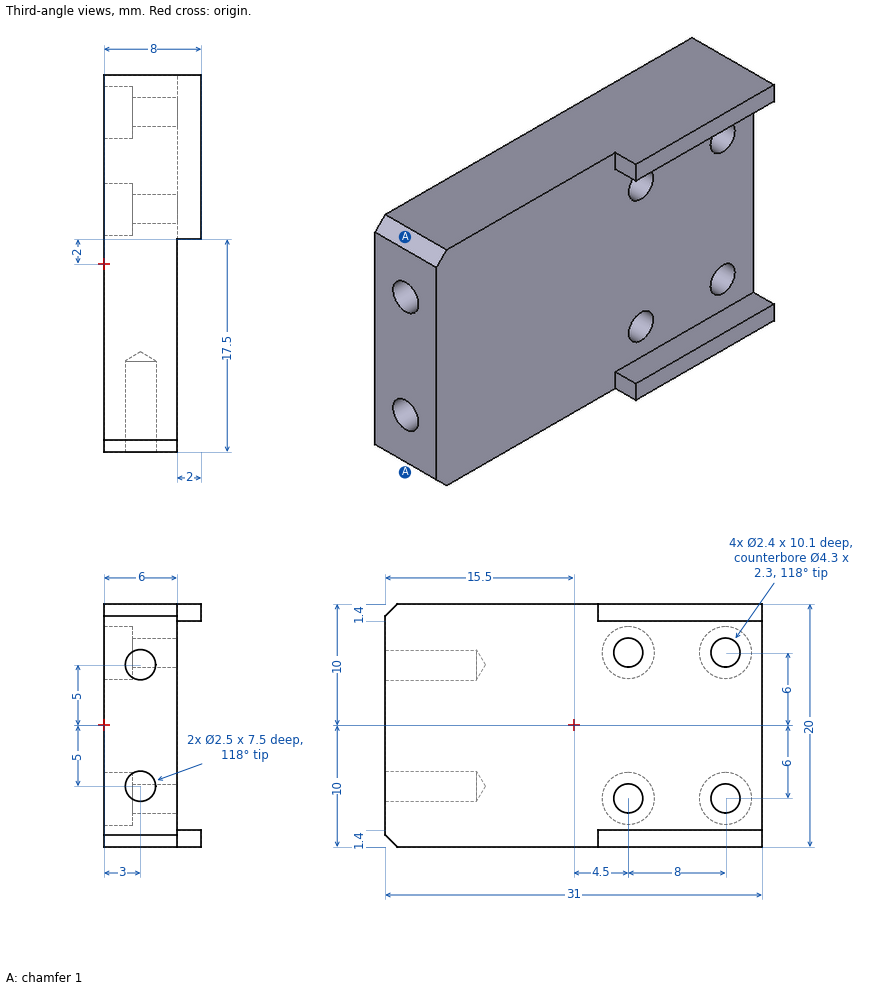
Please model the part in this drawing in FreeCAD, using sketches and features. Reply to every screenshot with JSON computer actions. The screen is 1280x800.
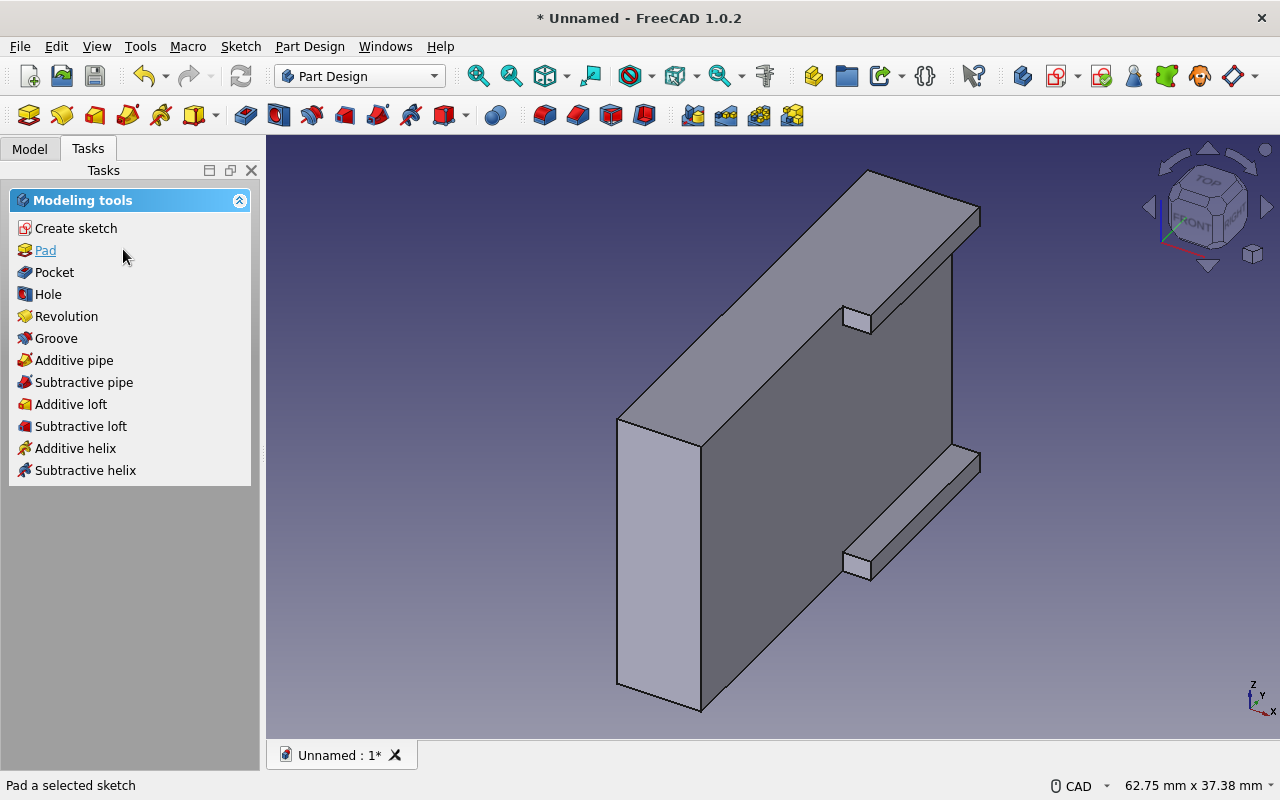
{"action": "left_click", "coordinate": [279, 116]}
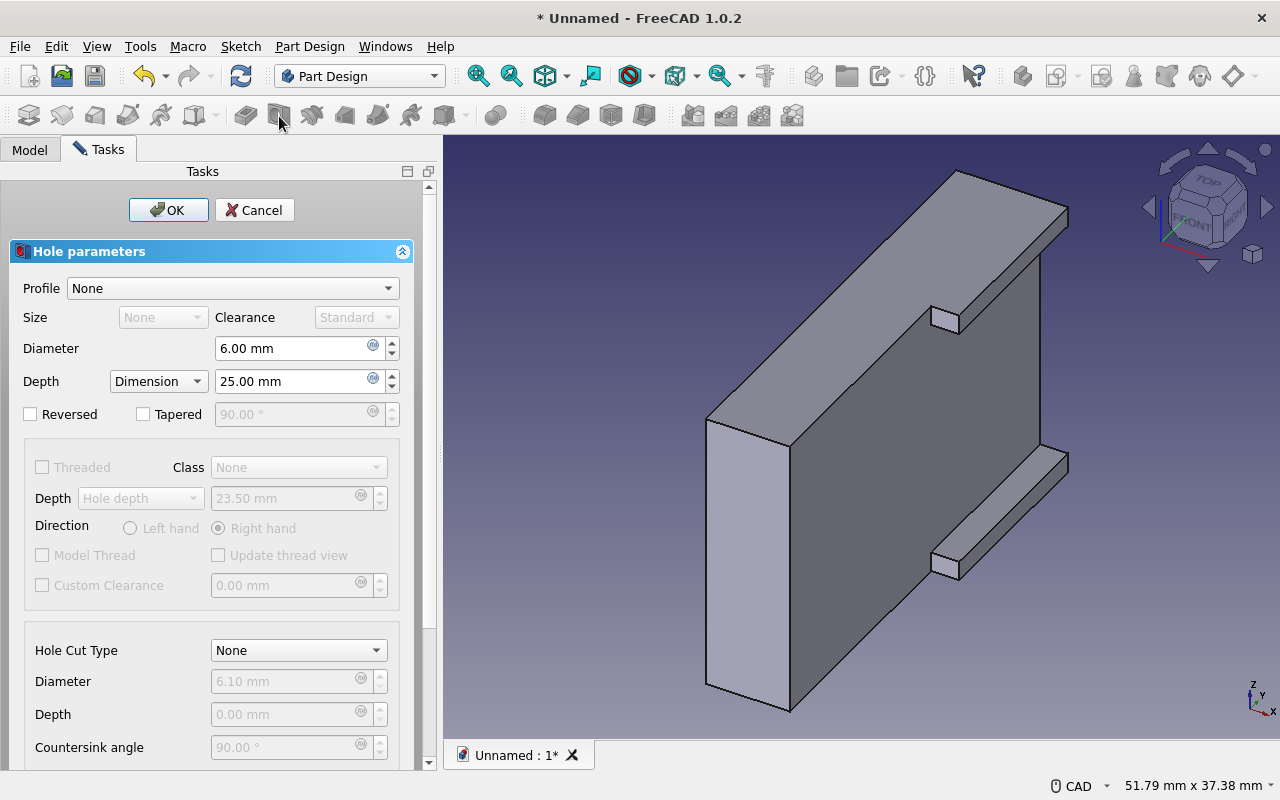
{"action": "triple_click", "coordinate": [300, 348]}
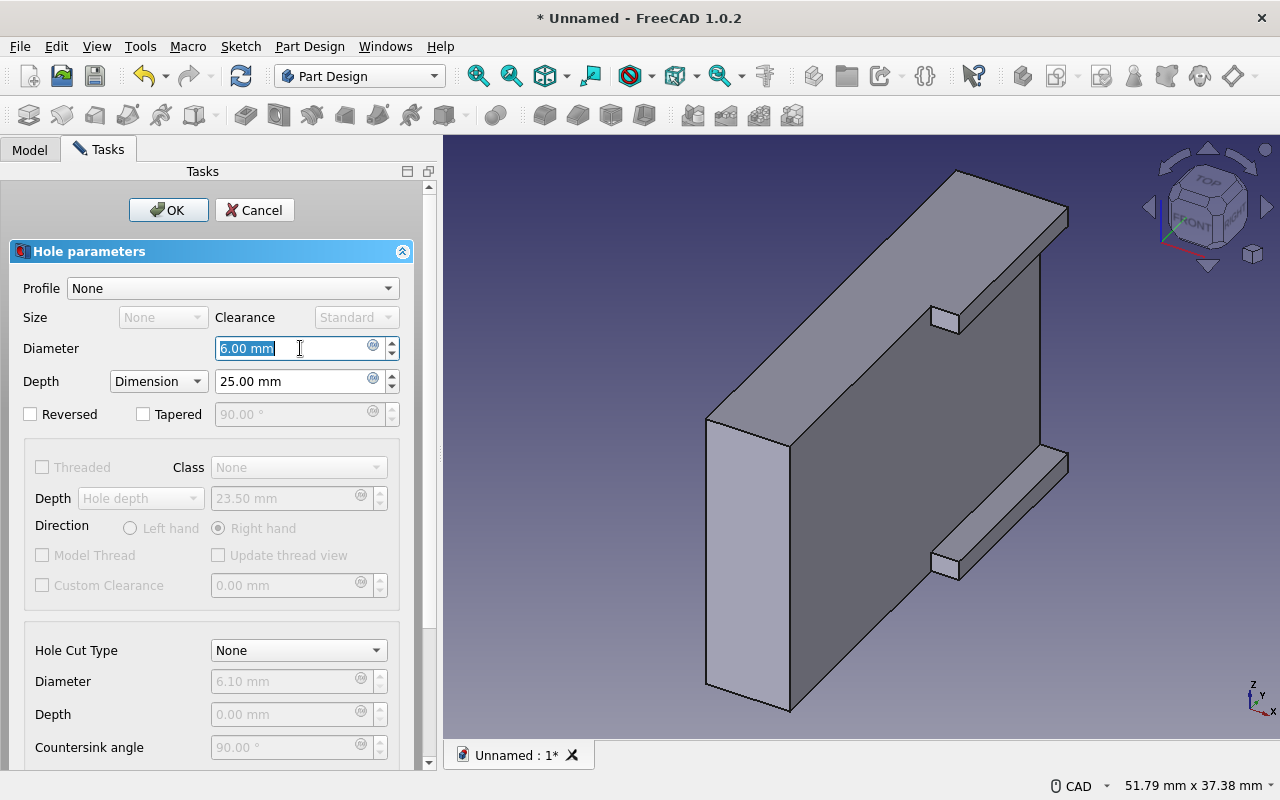
{"action": "type", "text": "2.4"}
{"action": "key", "text": "Tab"}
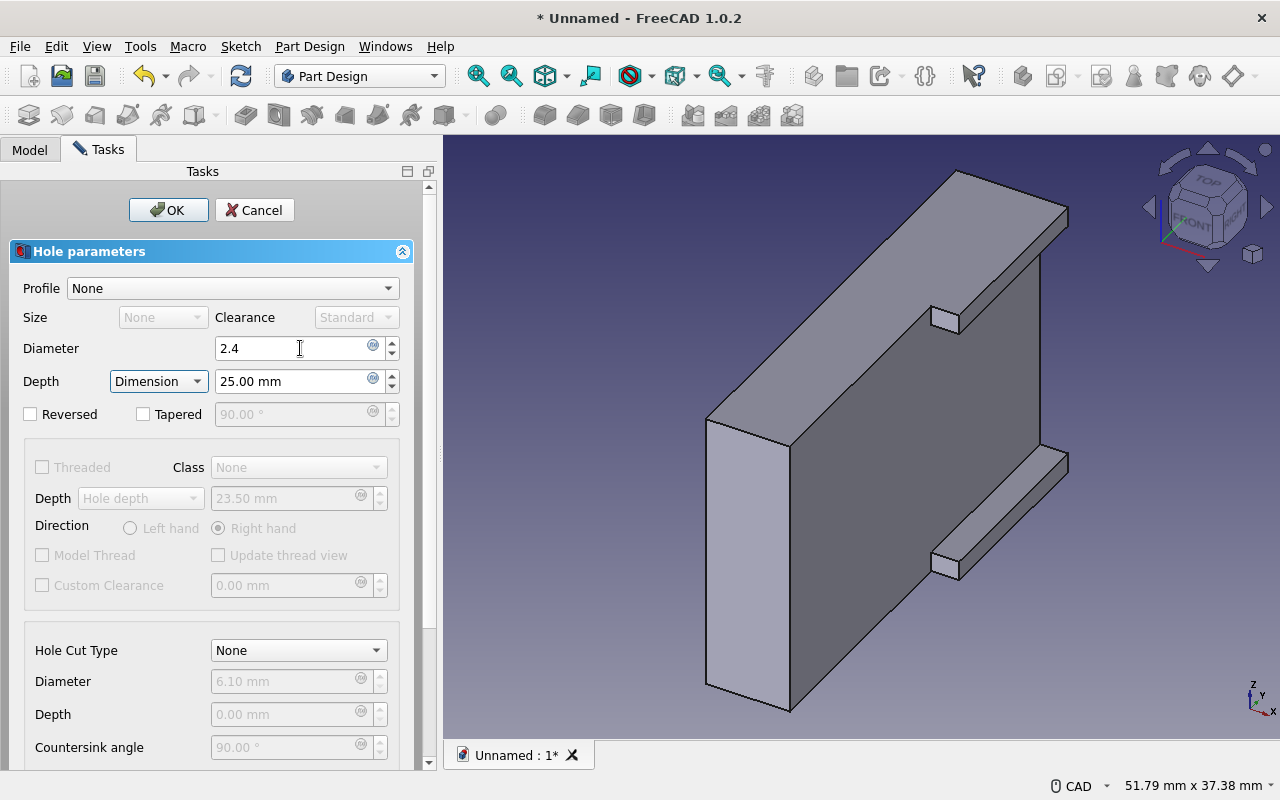
{"action": "triple_click", "coordinate": [300, 382]}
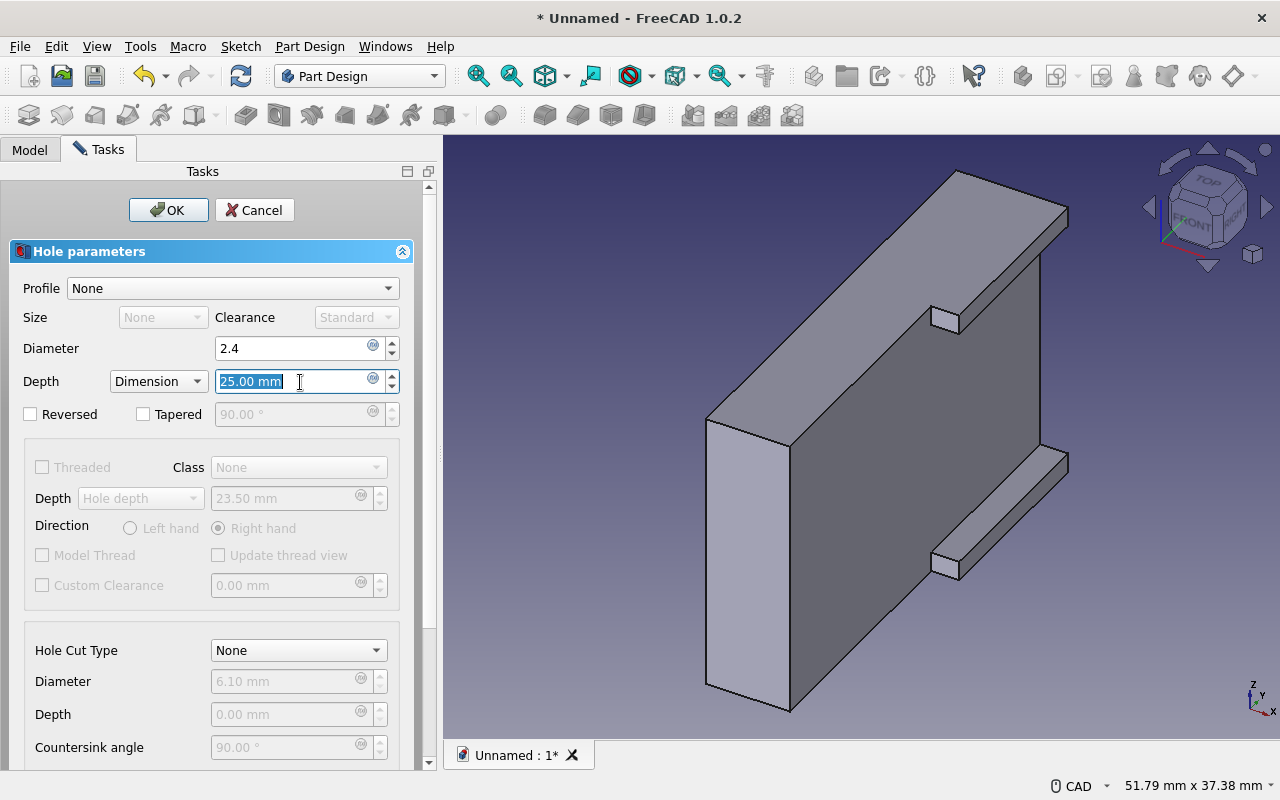
{"action": "type", "text": "10.1"}
{"action": "key", "text": "Tab"}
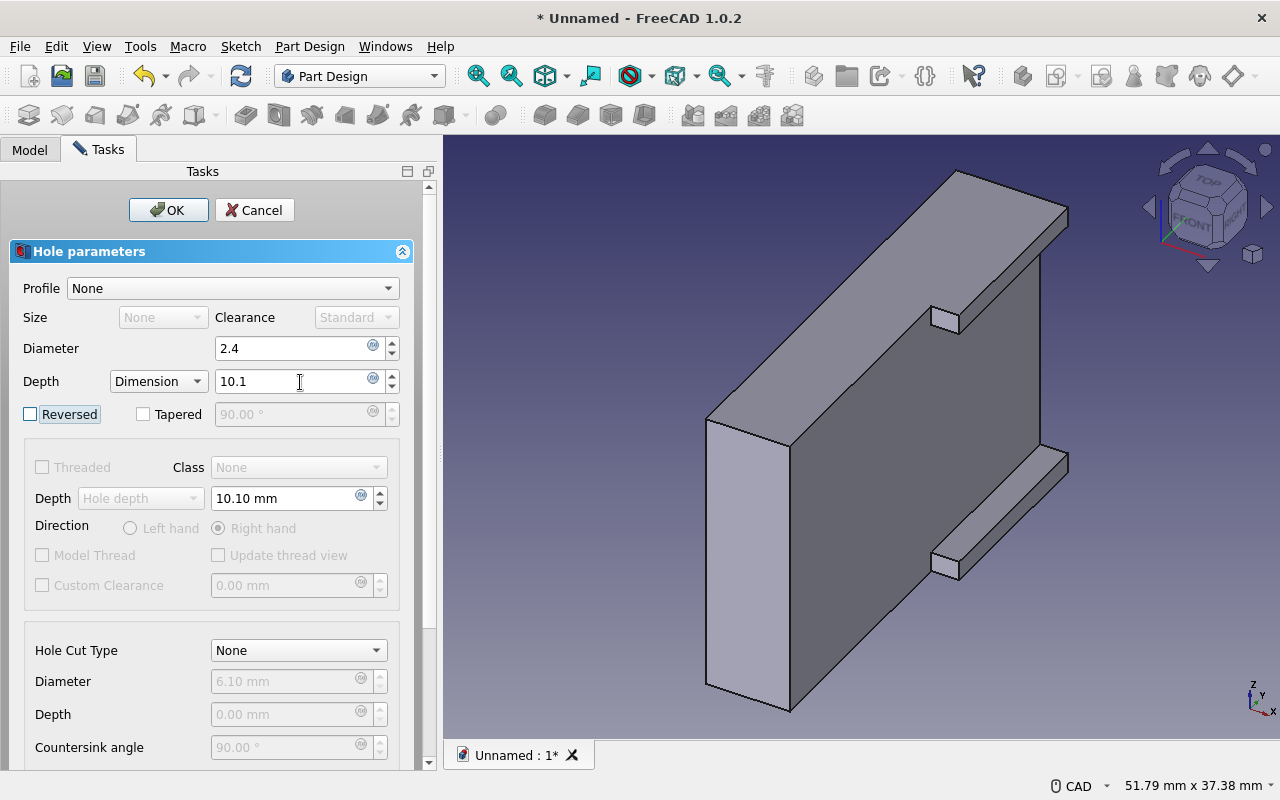
{"action": "left_click", "coordinate": [31, 414]}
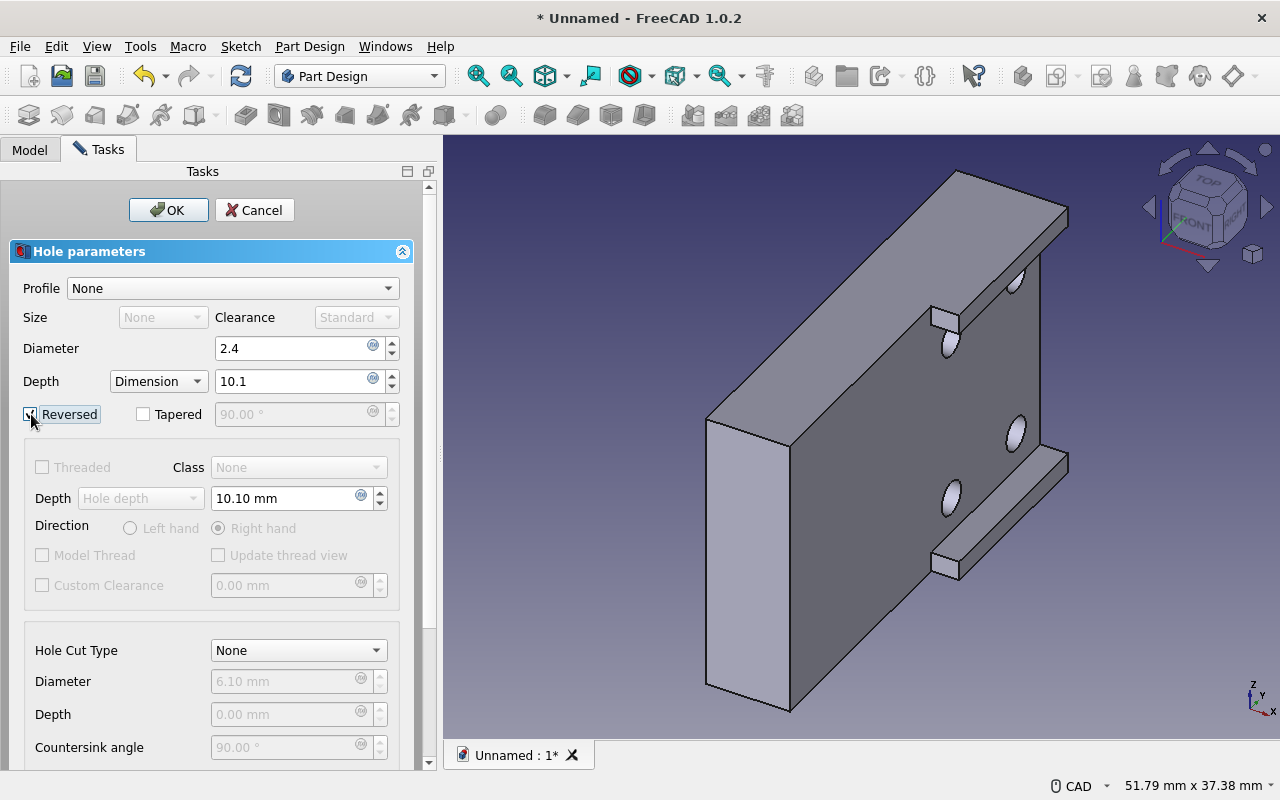
{"action": "left_click", "coordinate": [300, 650]}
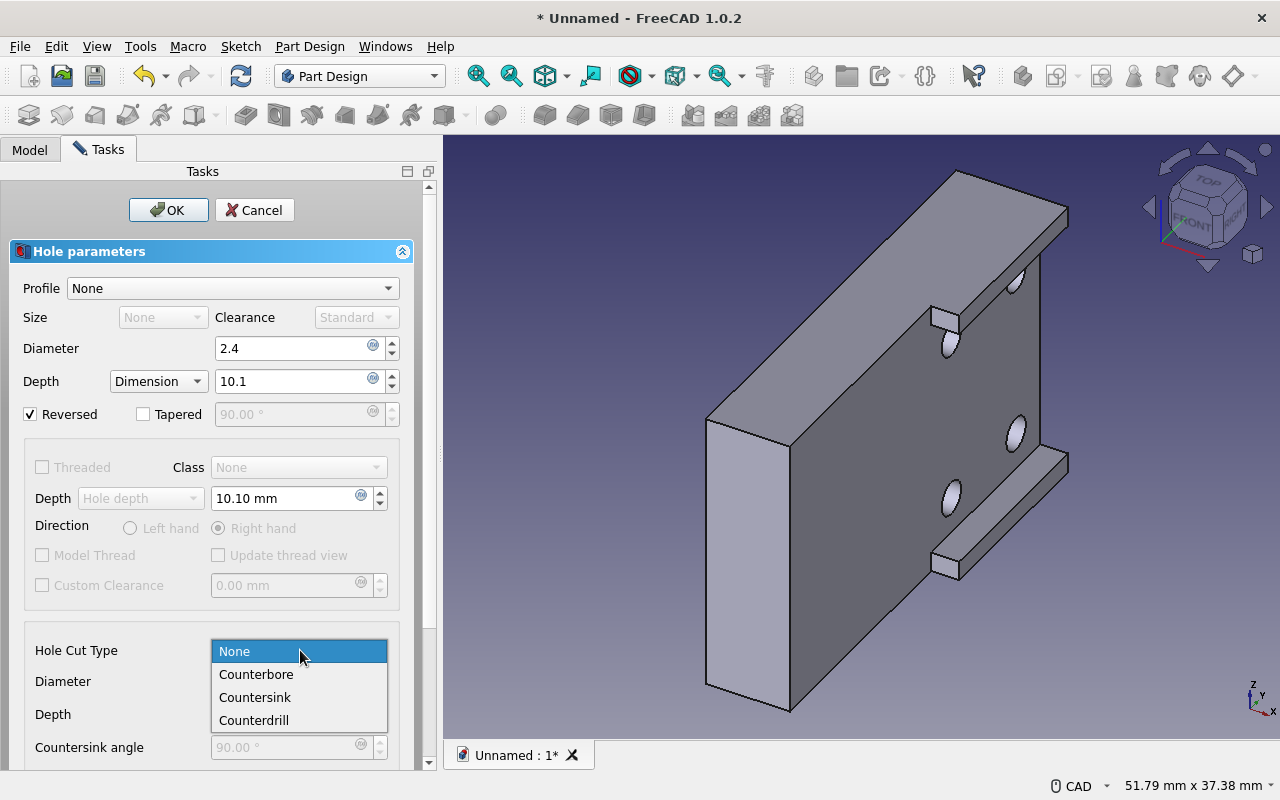
{"action": "left_click", "coordinate": [298, 674]}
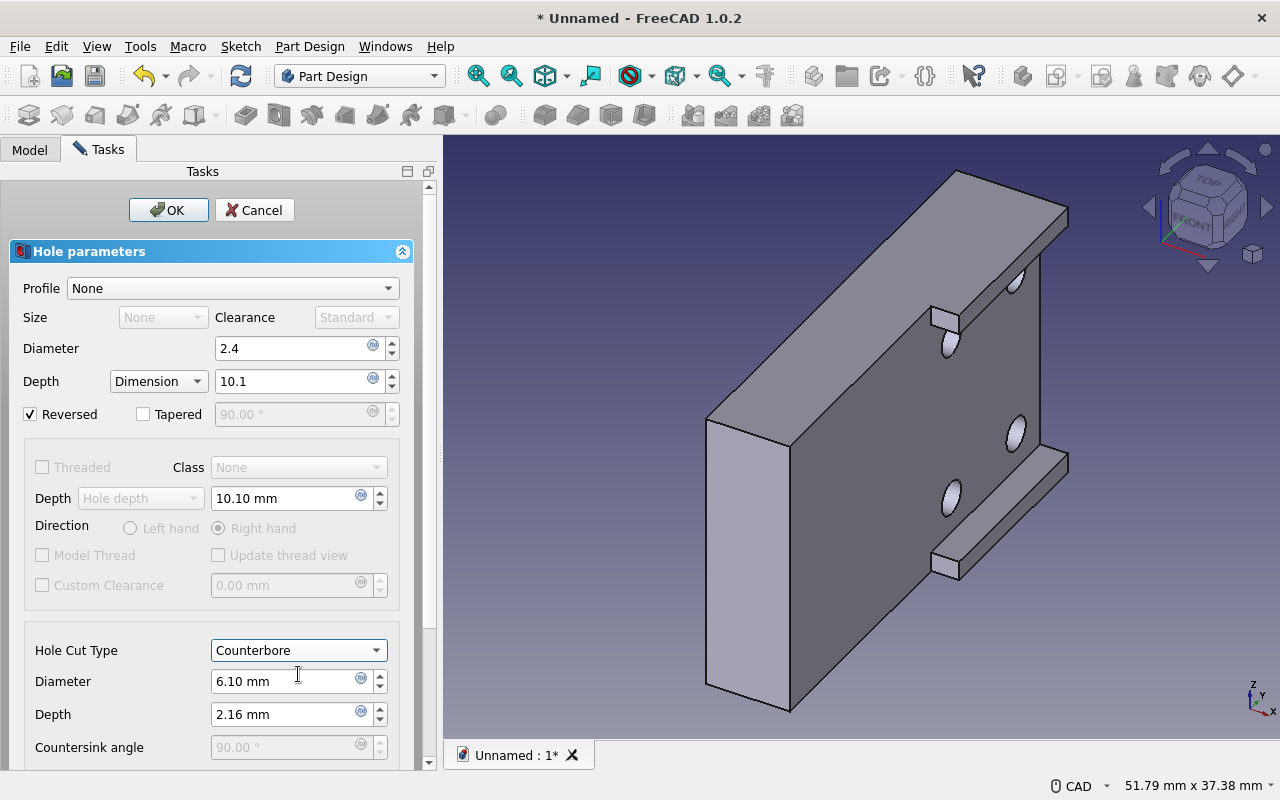
{"action": "triple_click", "coordinate": [292, 682]}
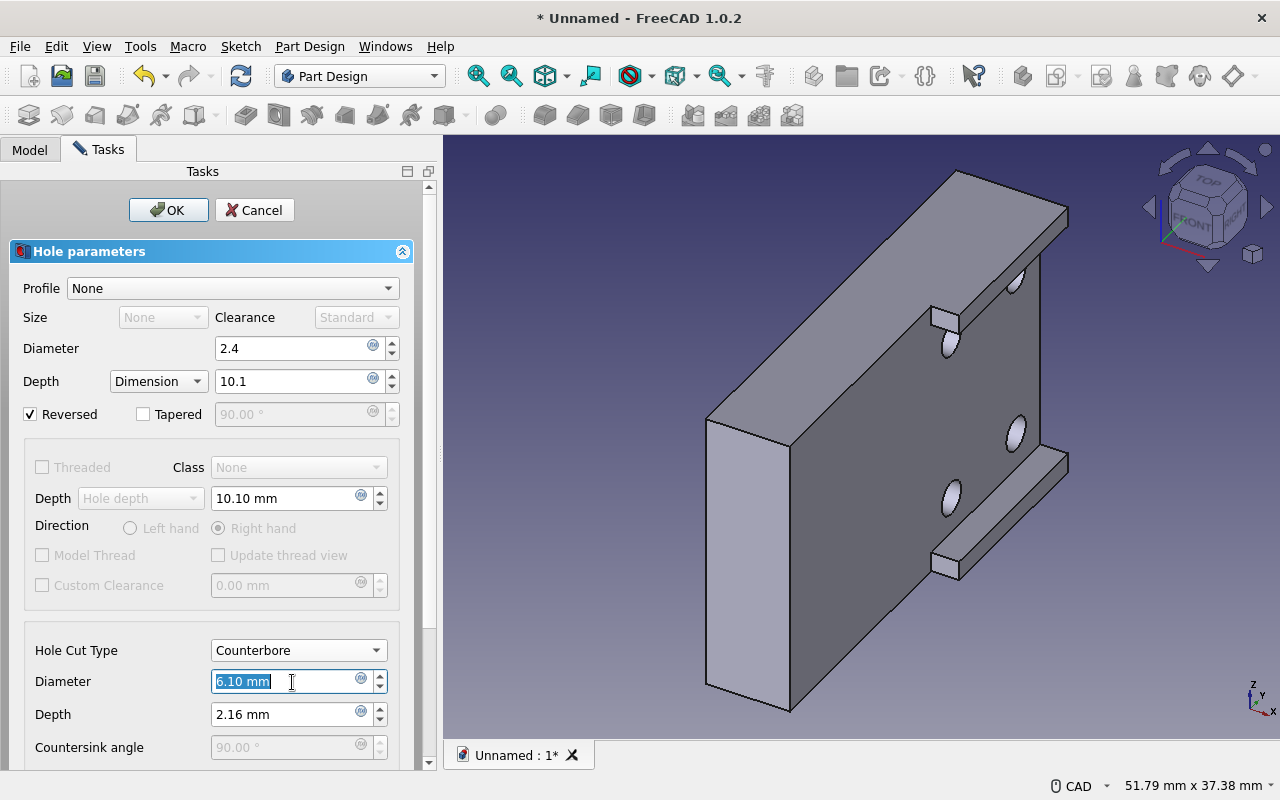
{"action": "type", "text": "4.3"}
{"action": "key", "text": "Tab"}